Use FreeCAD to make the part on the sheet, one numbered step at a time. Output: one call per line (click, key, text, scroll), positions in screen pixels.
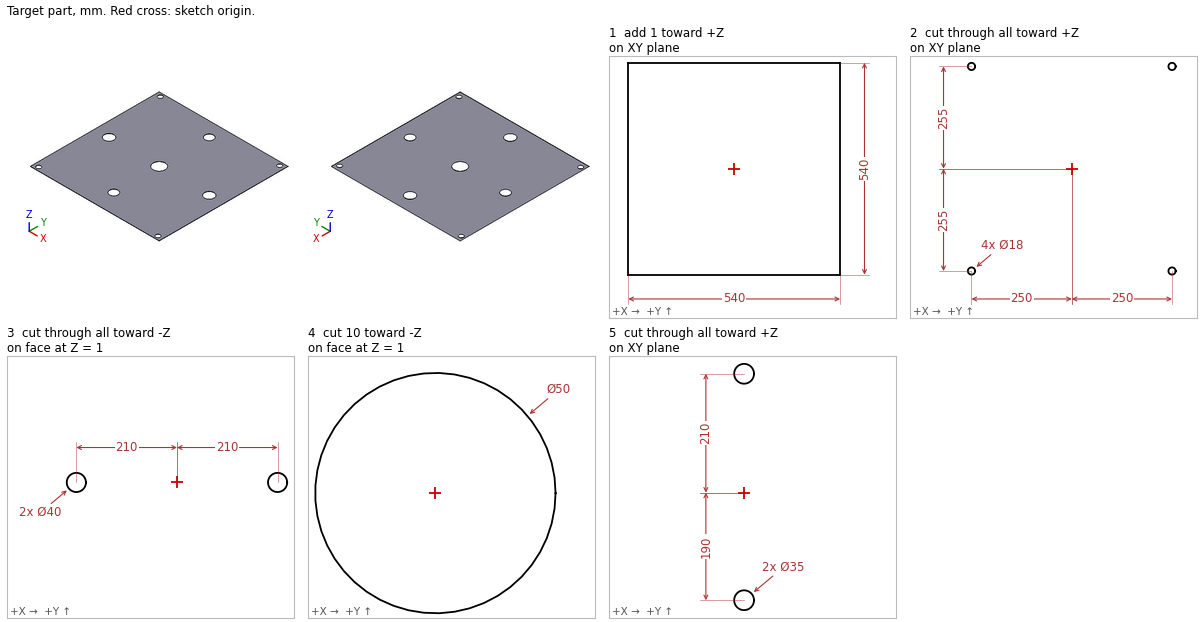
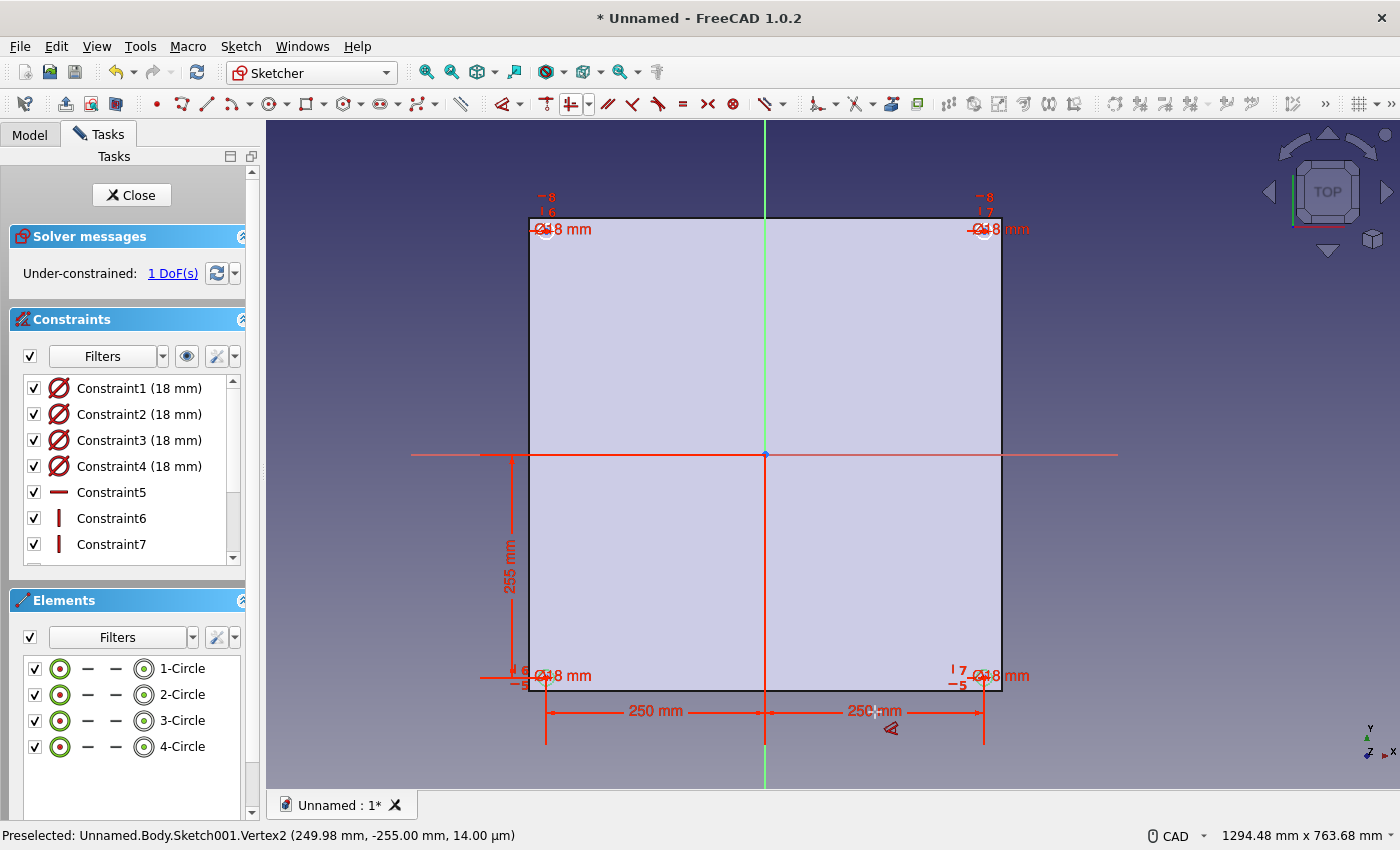
click(546, 231)
click(512, 343)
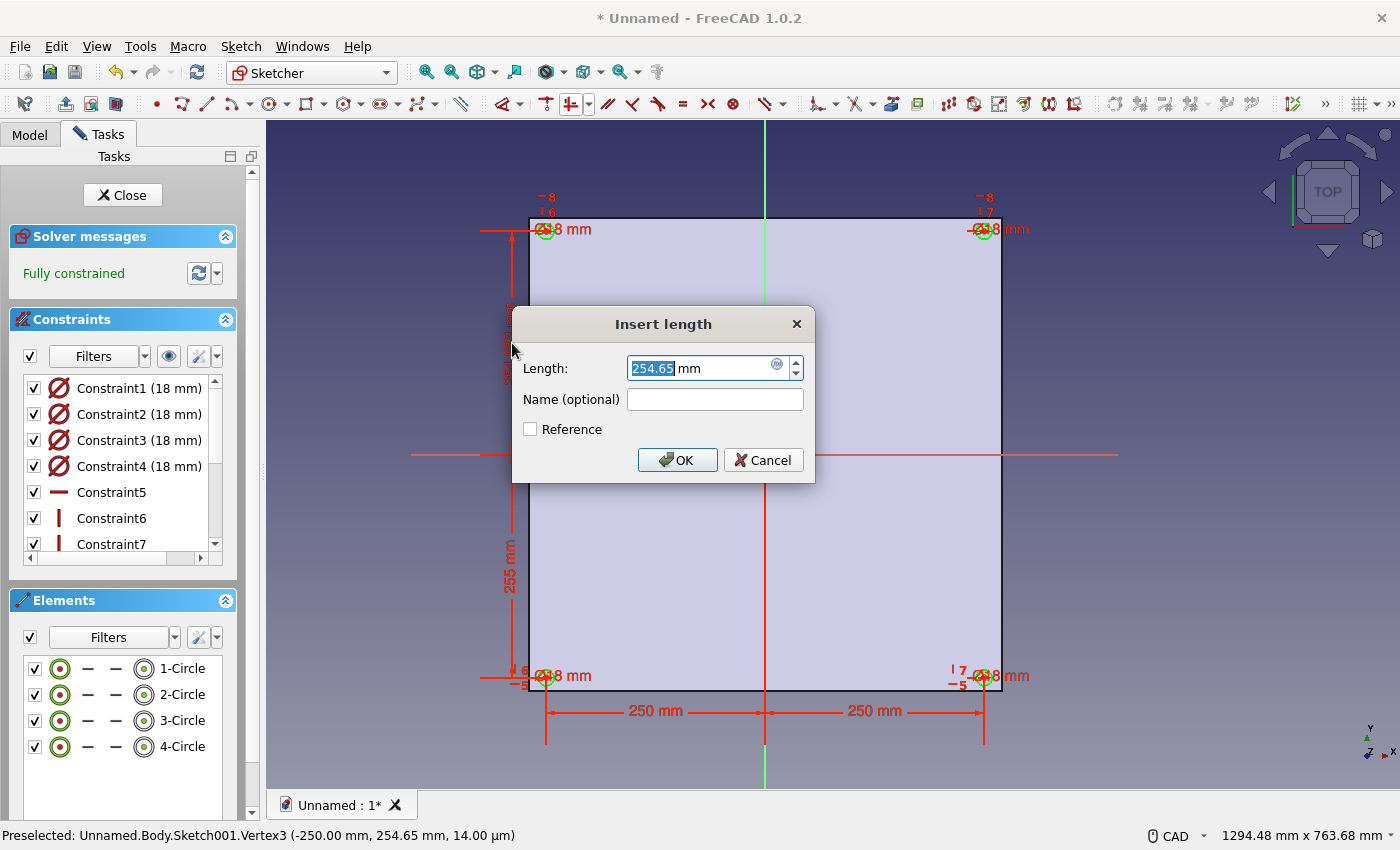
text(255)
key(Return)
key(Escape)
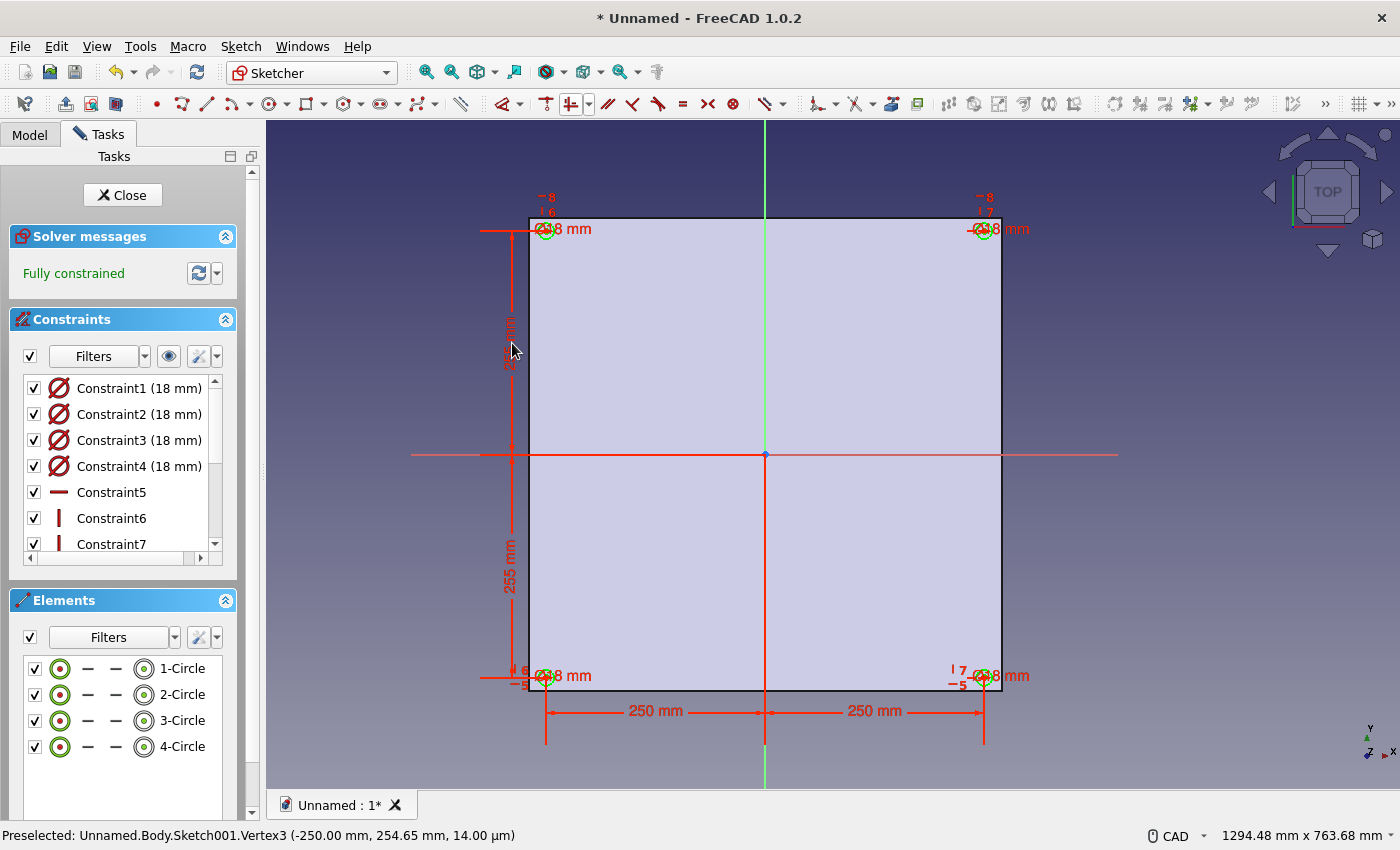
click(123, 195)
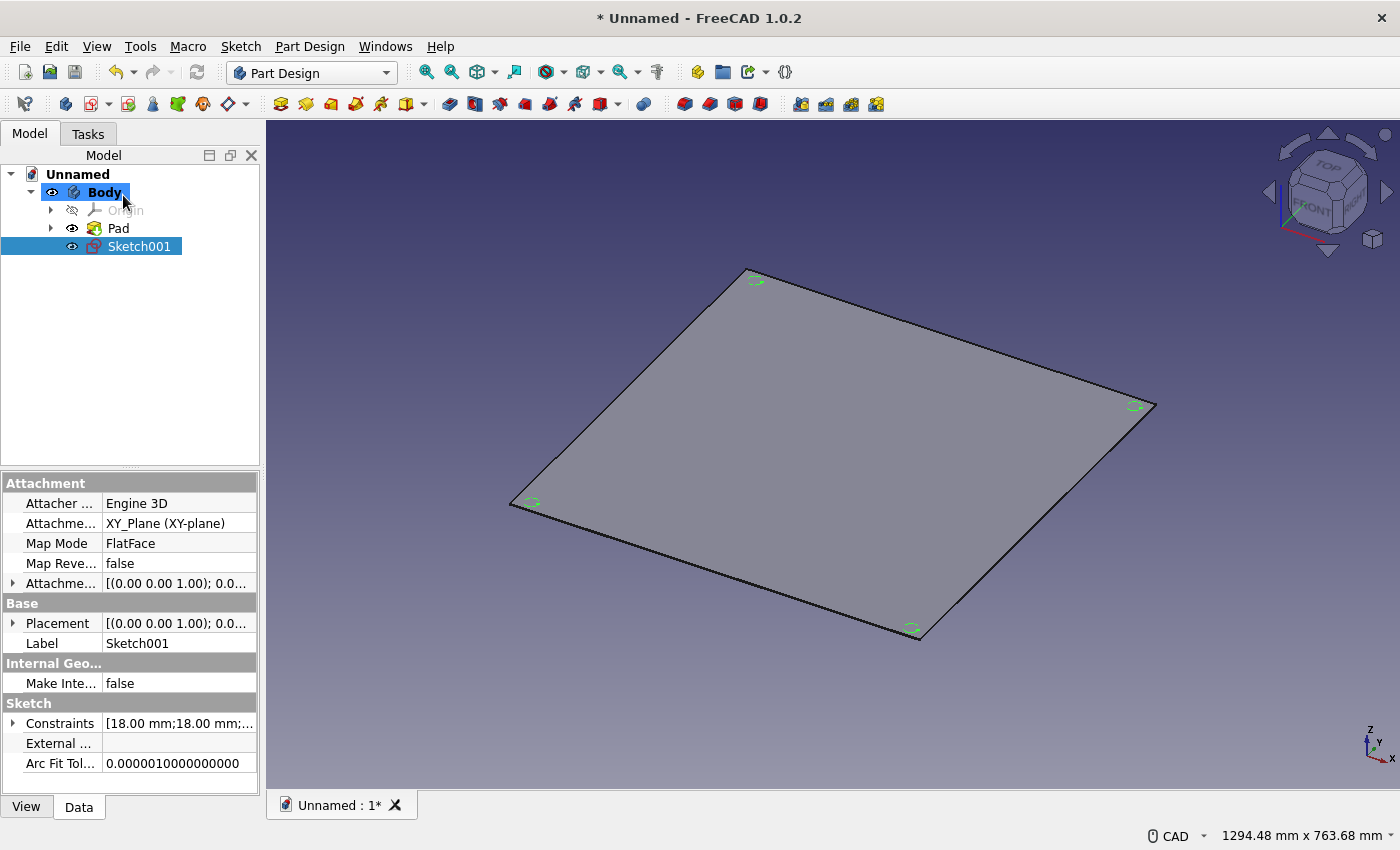
click(450, 104)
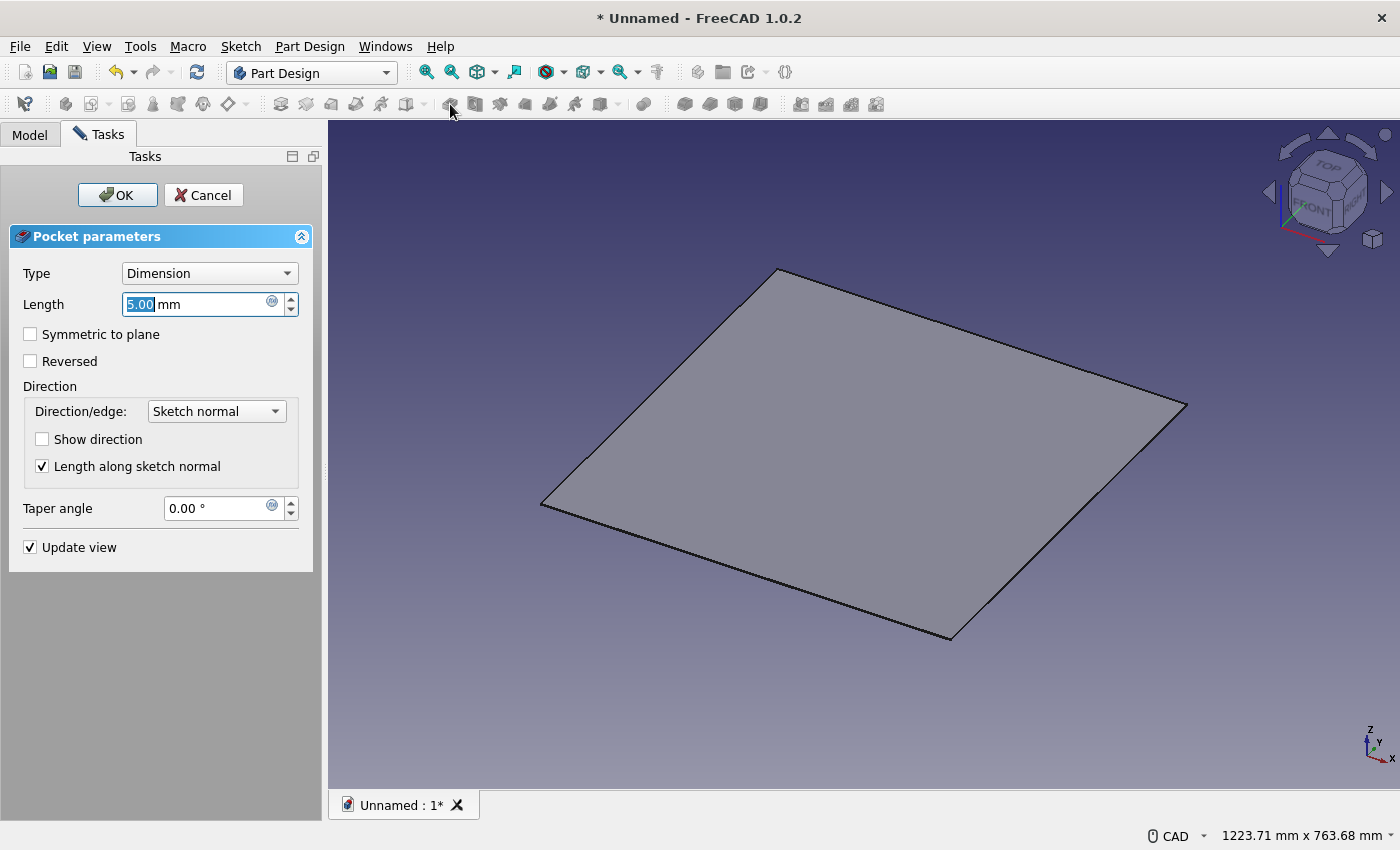
click(210, 274)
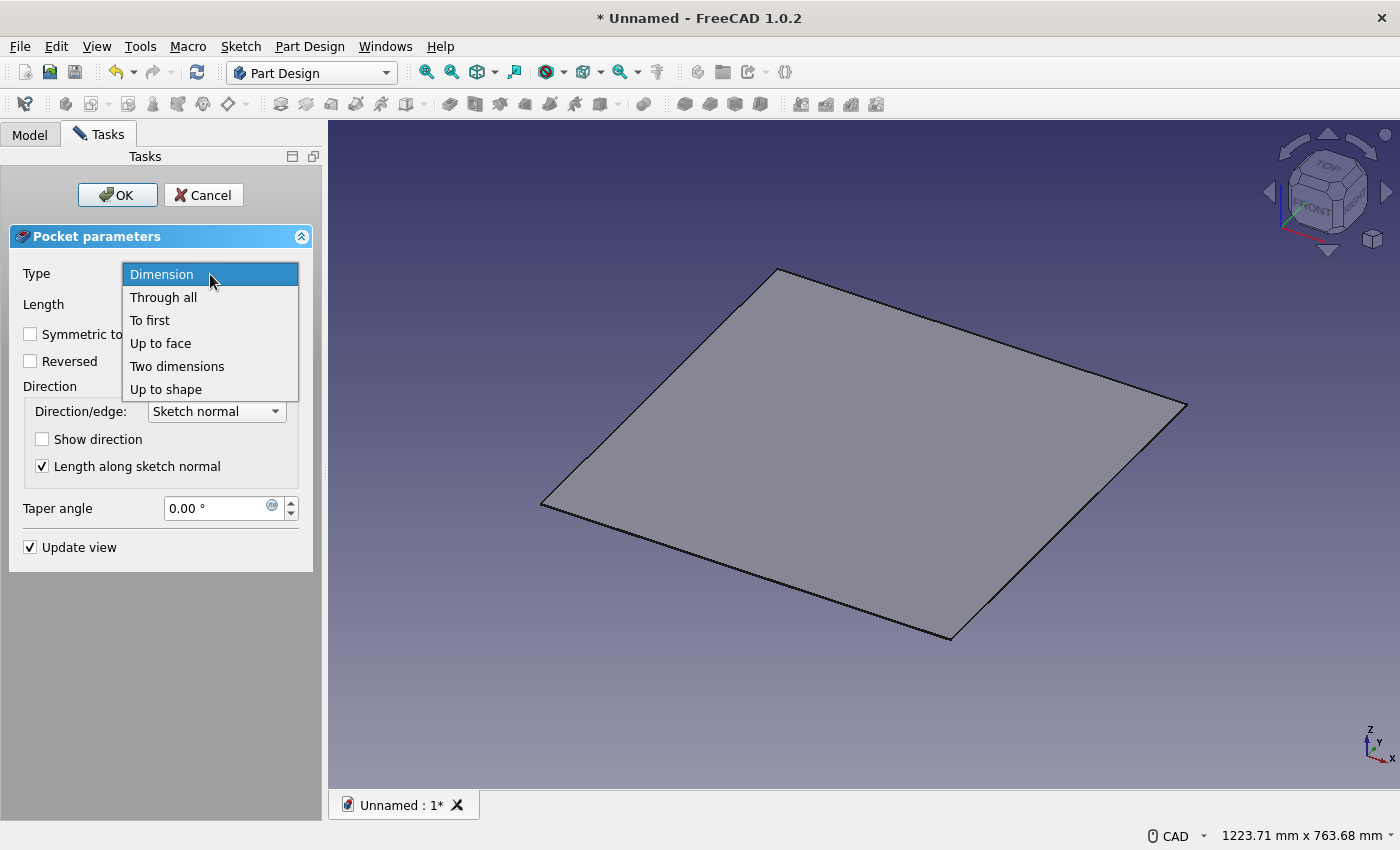
click(208, 298)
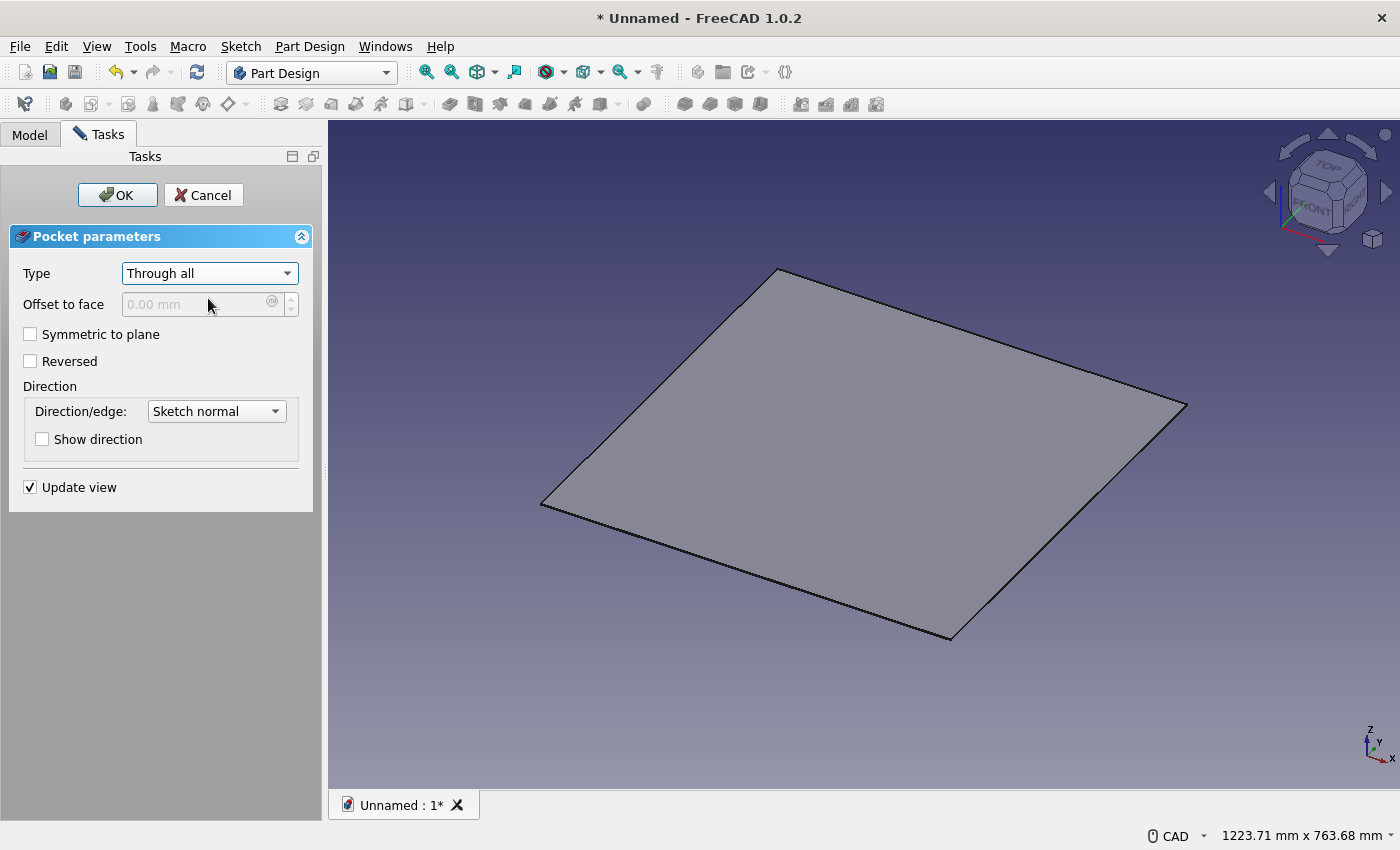
click(31, 361)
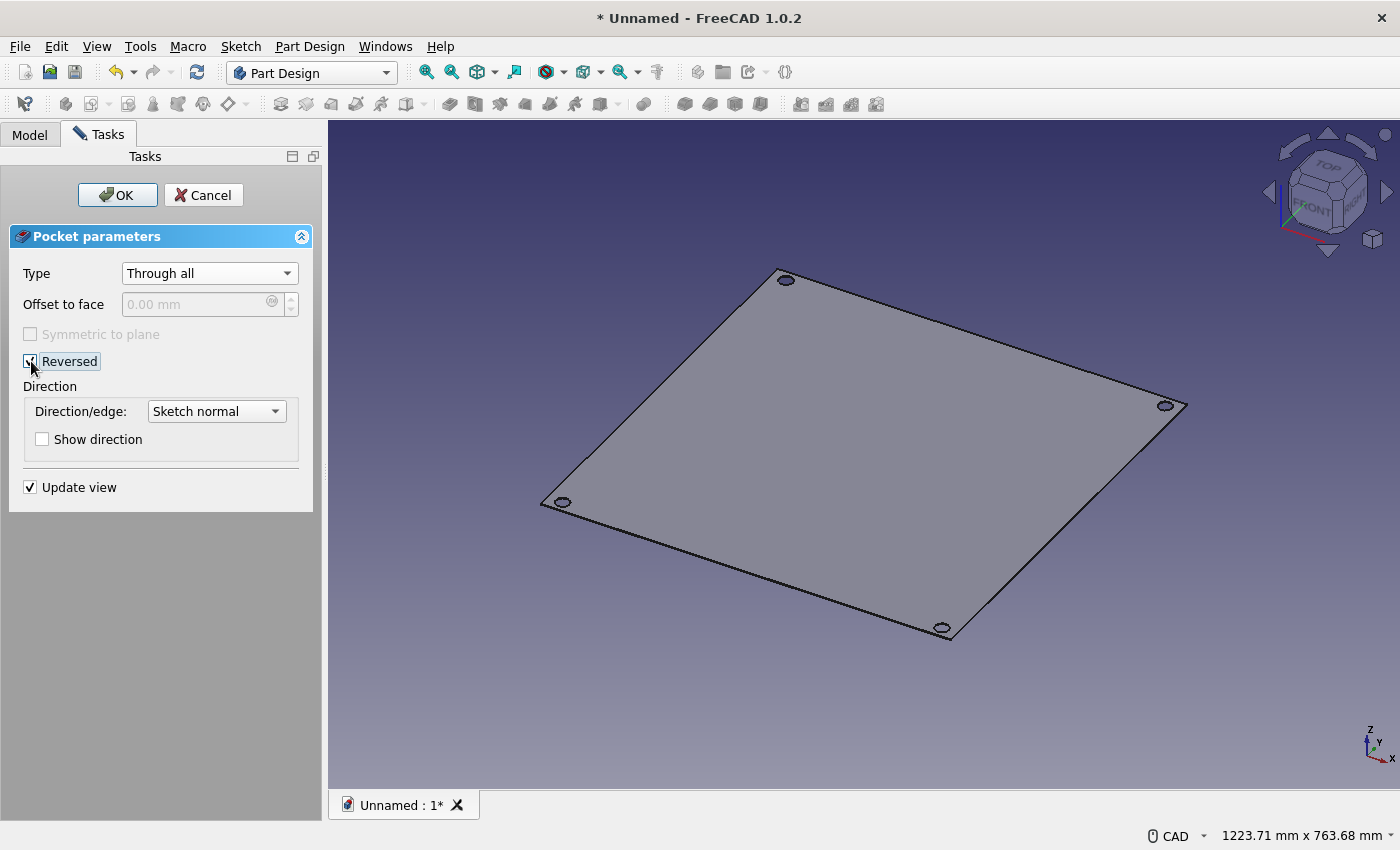
click(118, 195)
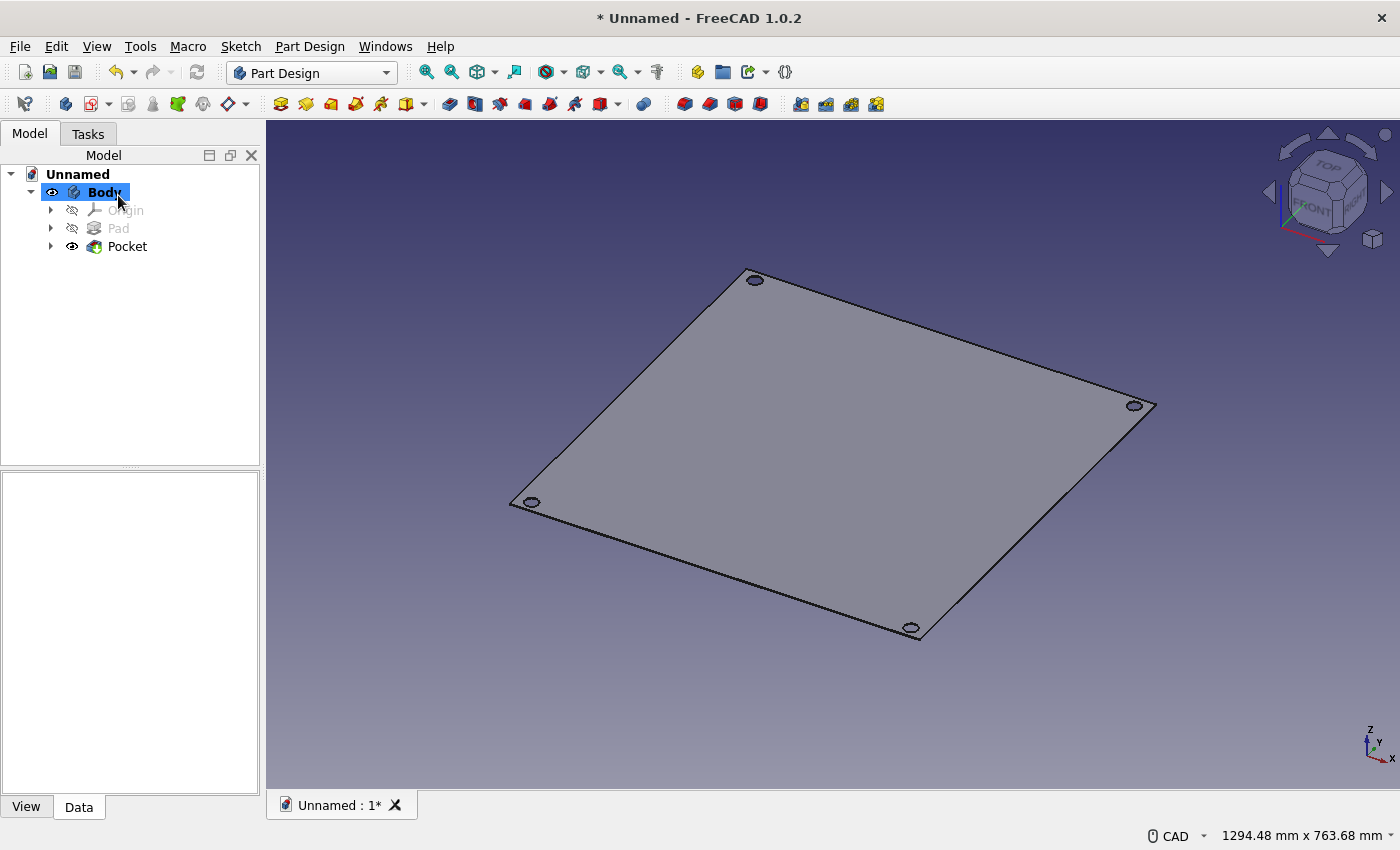
click(833, 453)